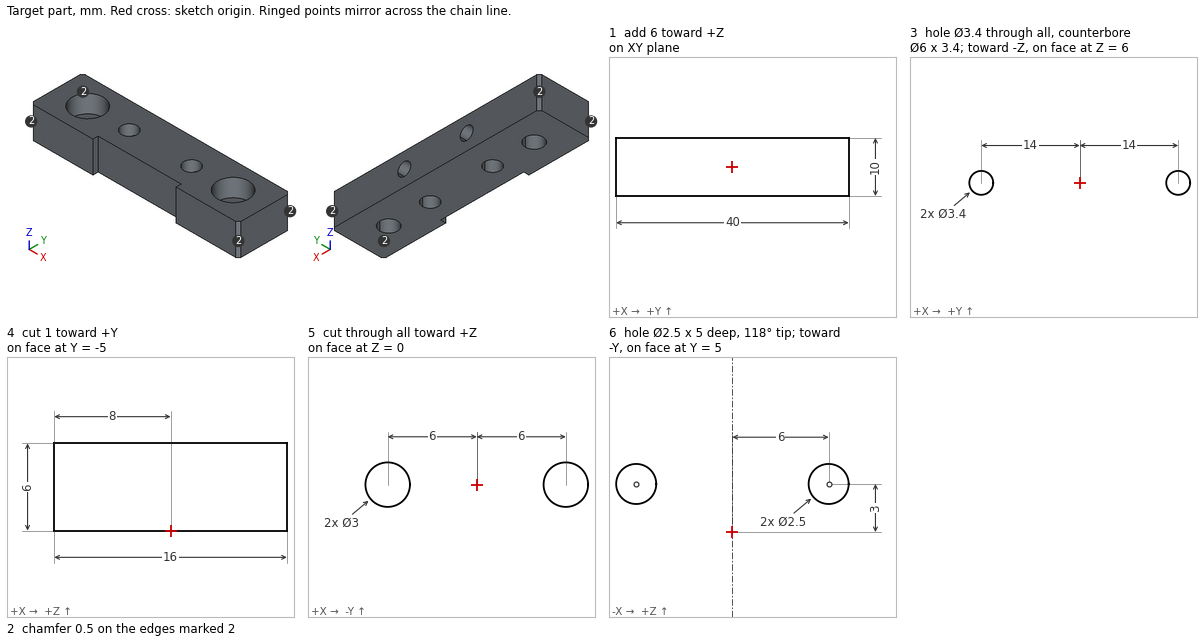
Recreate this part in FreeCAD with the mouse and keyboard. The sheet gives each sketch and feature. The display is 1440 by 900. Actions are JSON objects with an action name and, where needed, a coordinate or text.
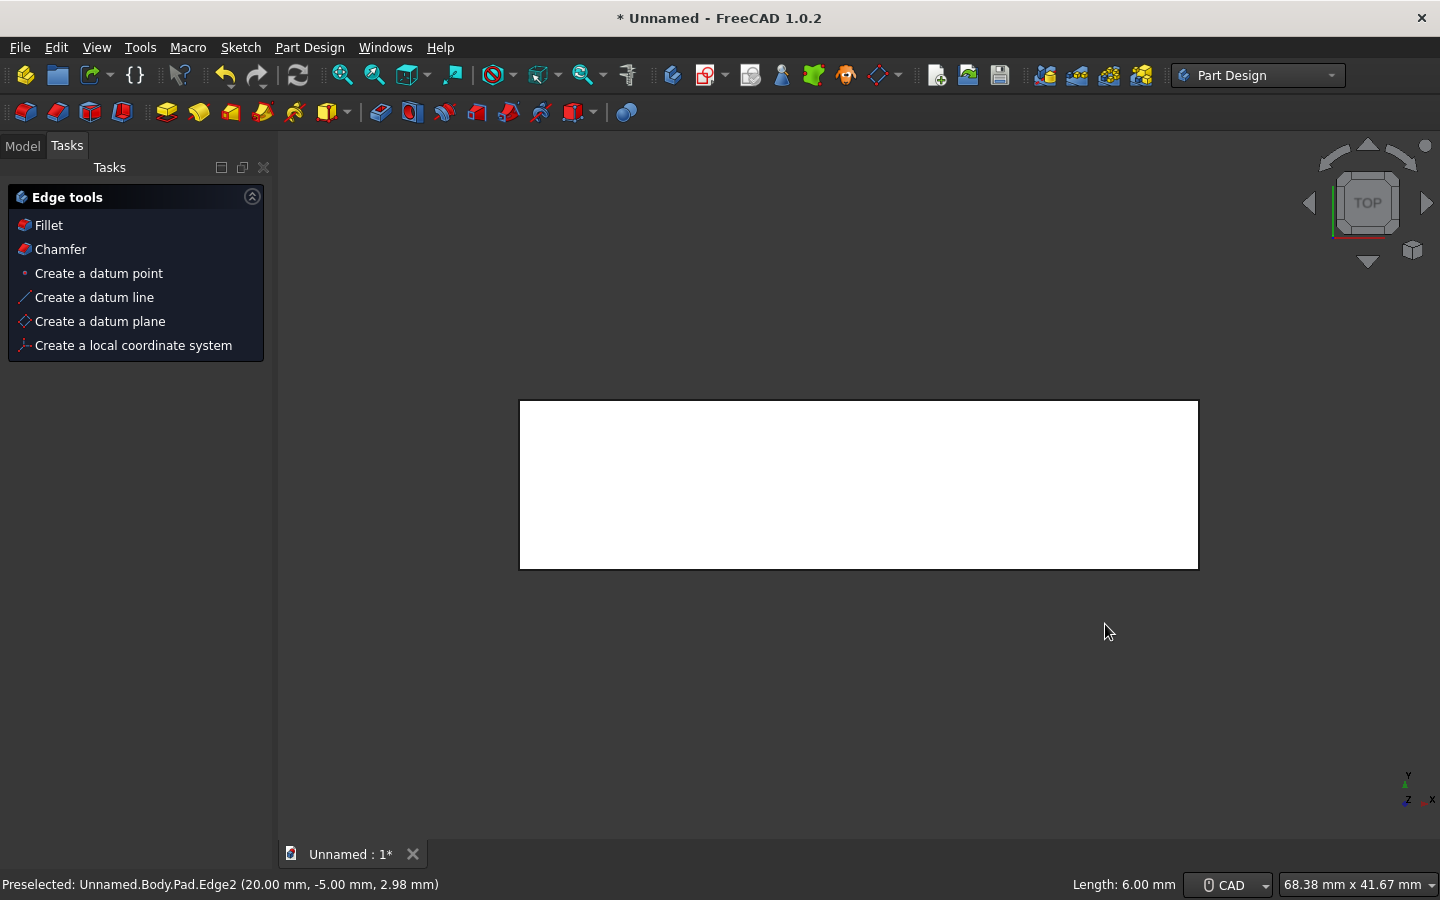
{"action": "key", "text": "1"}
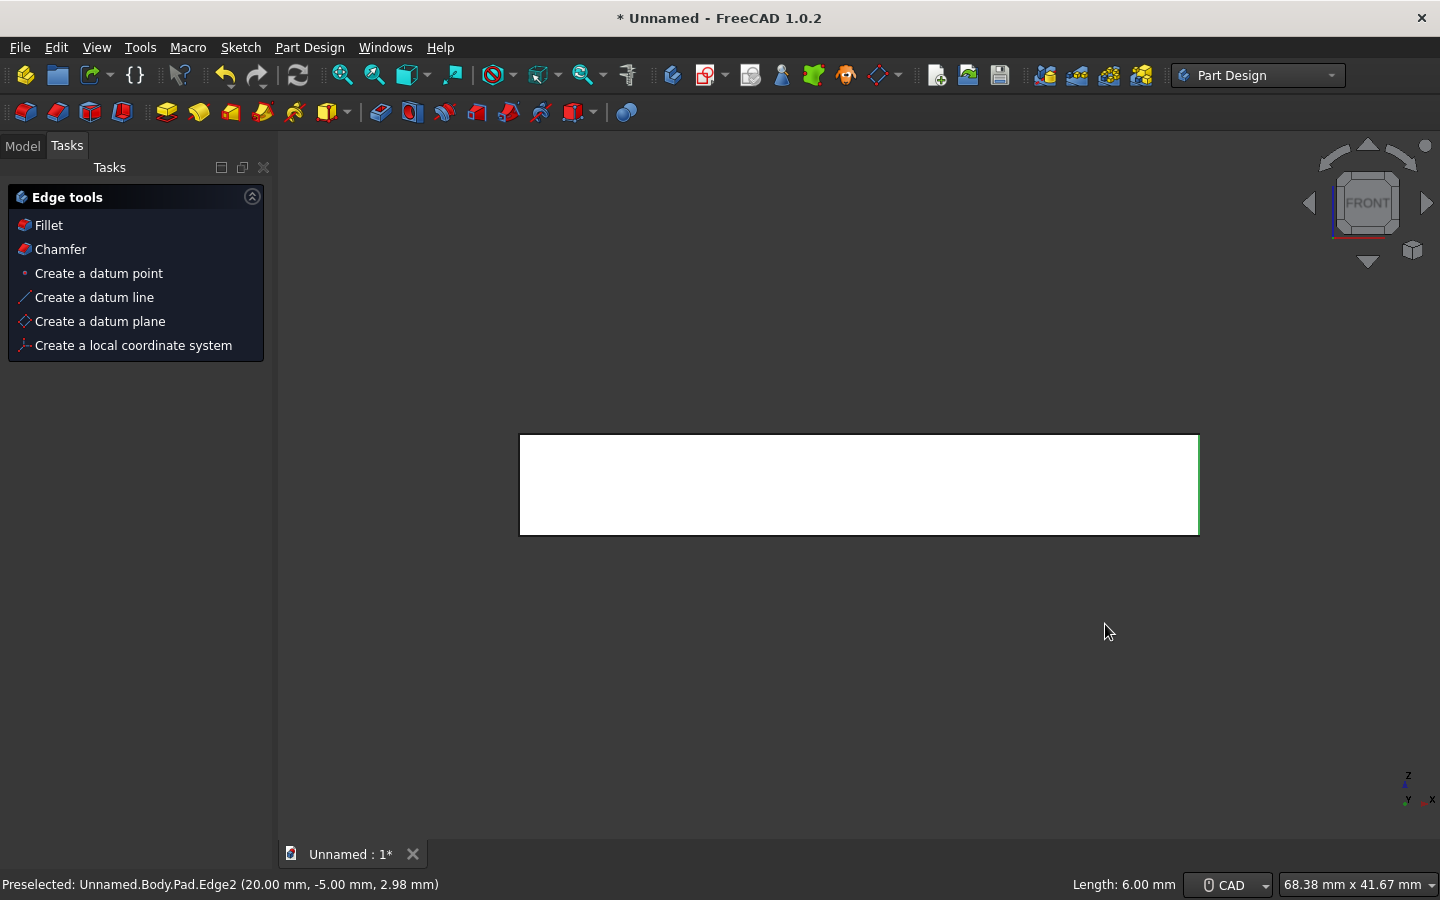
{"action": "left_click", "coordinate": [519, 484], "text": "ctrl"}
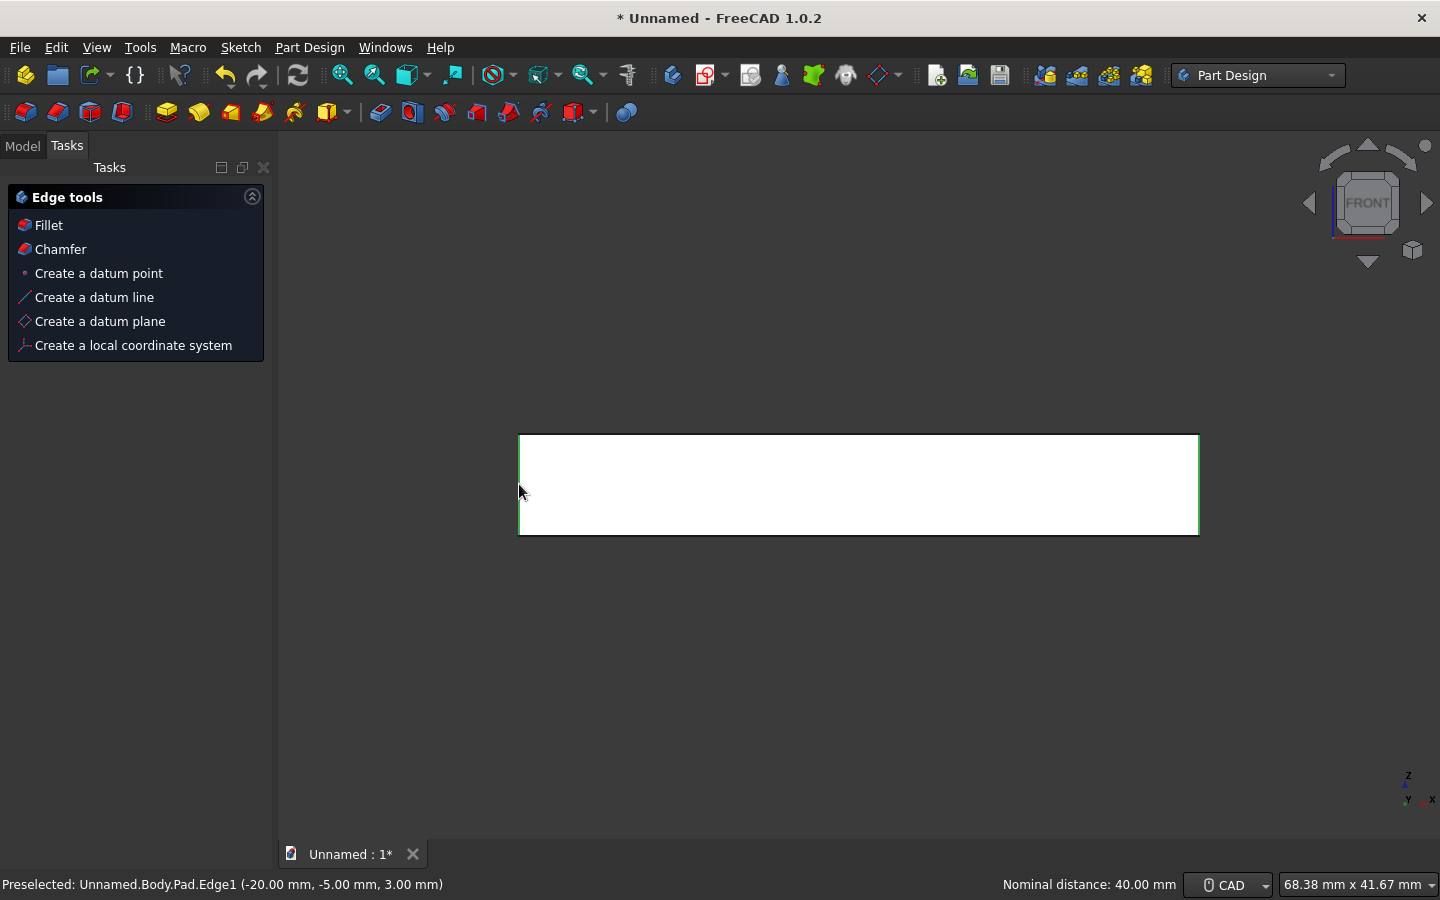
{"action": "key", "text": "3"}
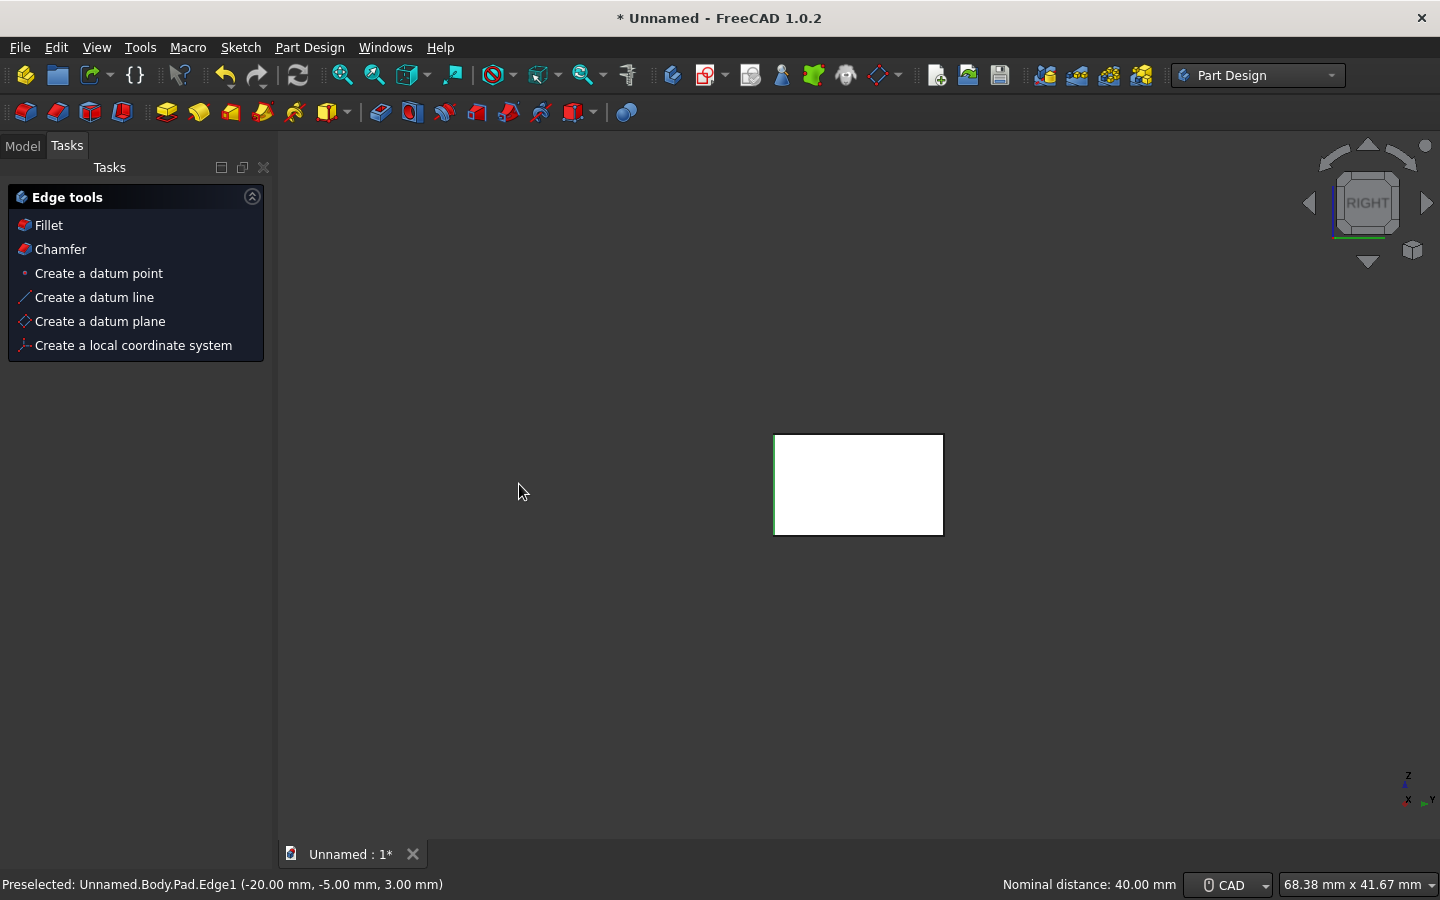
{"action": "left_click", "coordinate": [344, 76]}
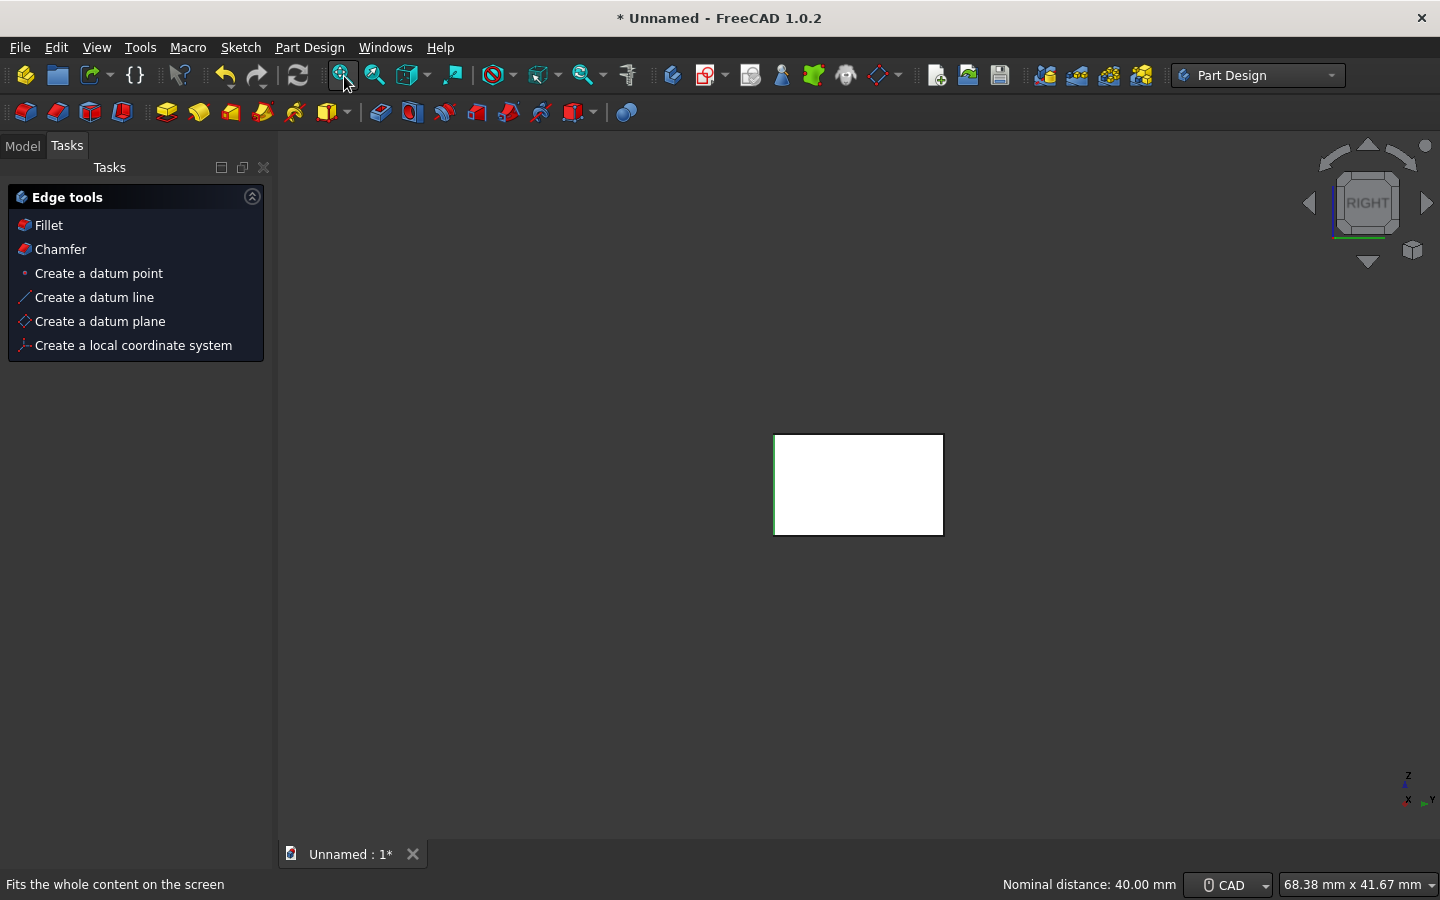
{"action": "left_click", "coordinate": [944, 484], "text": "ctrl"}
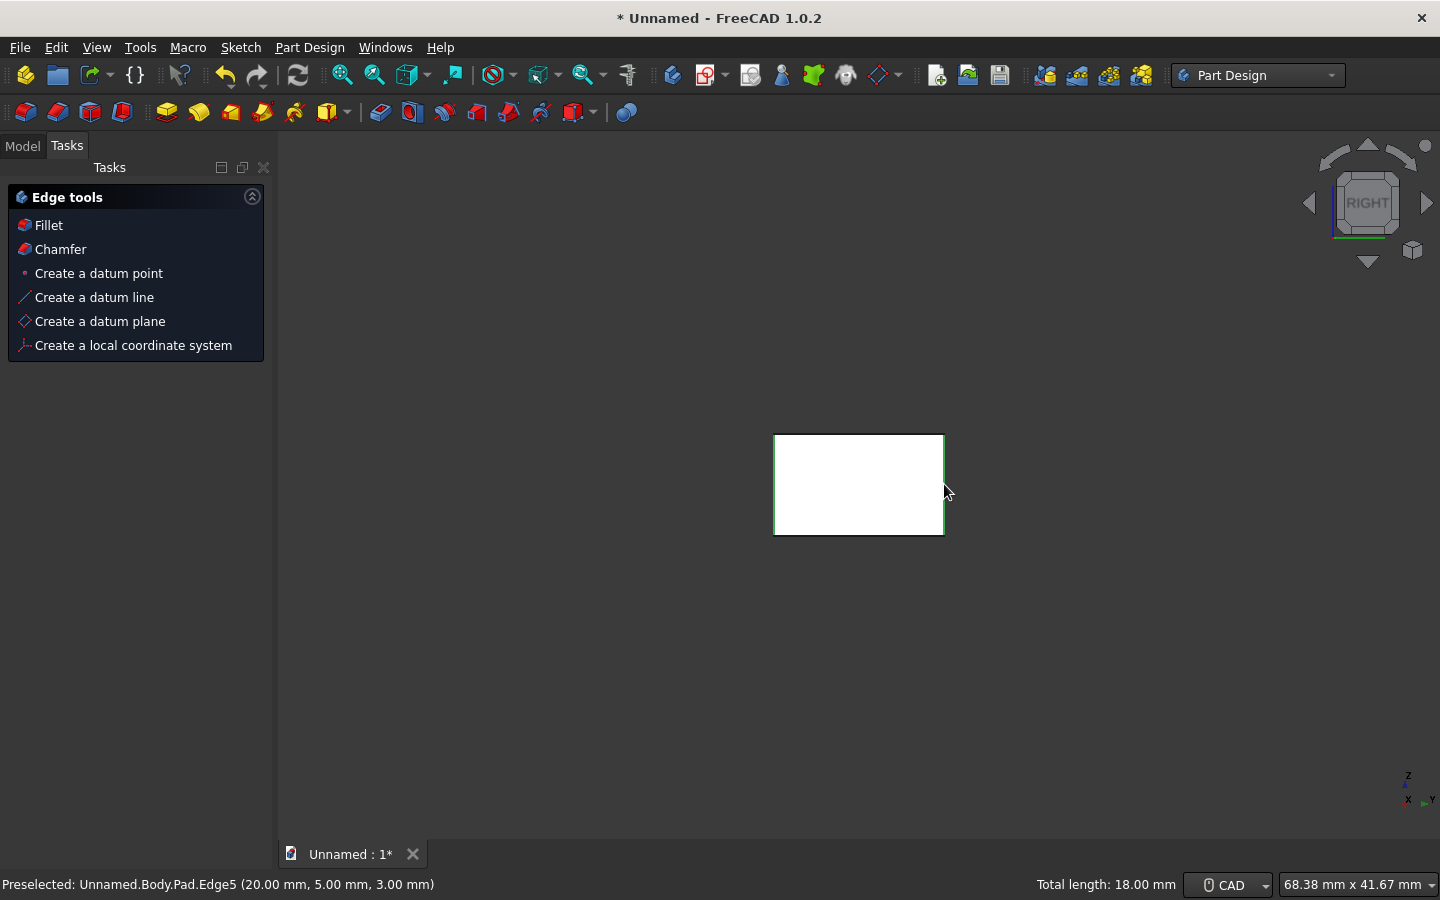
{"action": "key", "text": "5"}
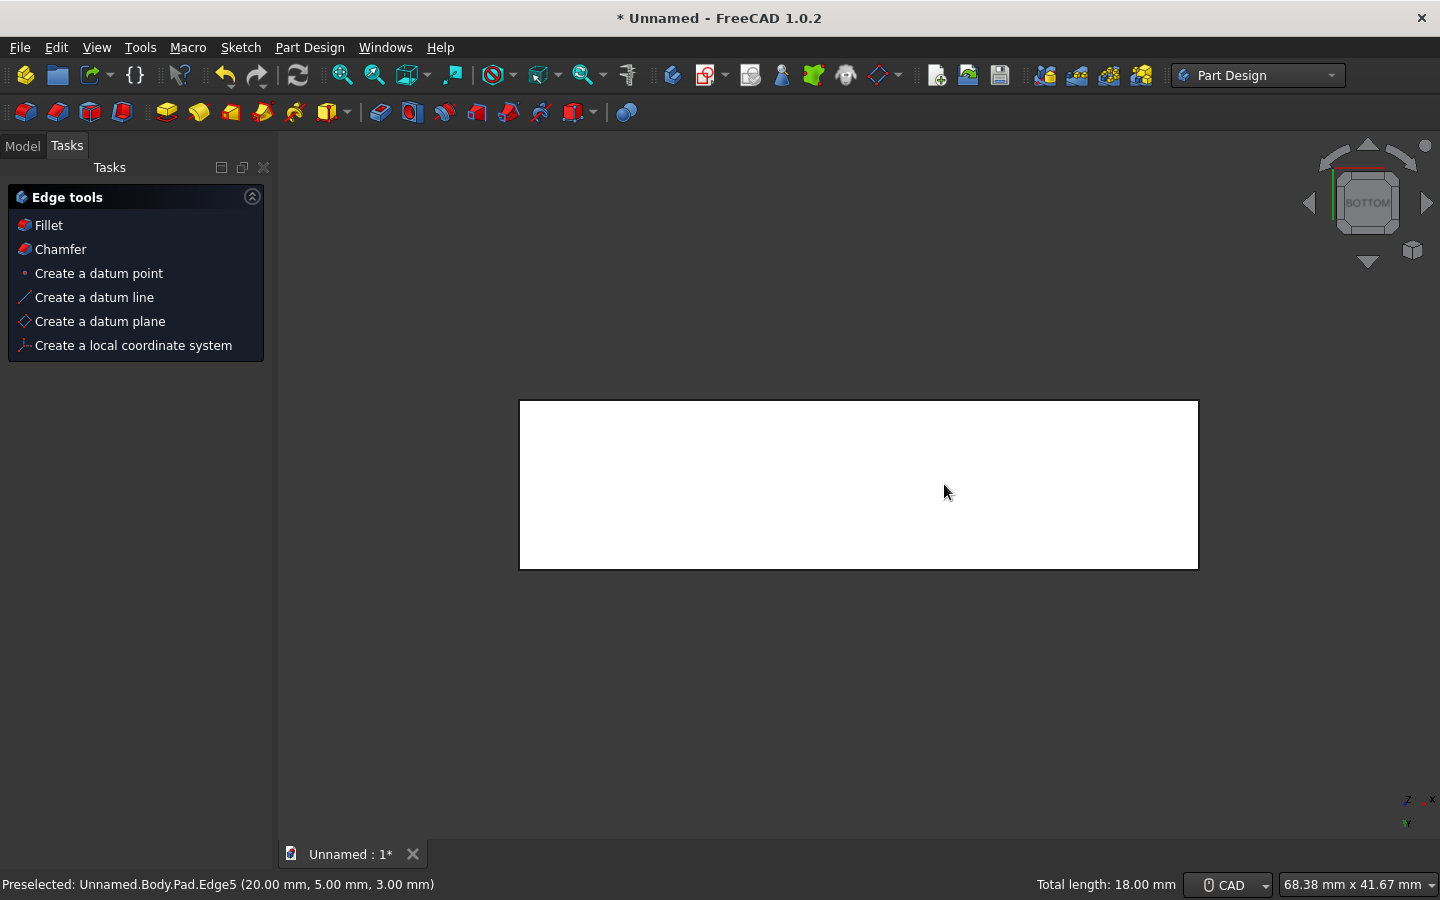
{"action": "key", "text": "4"}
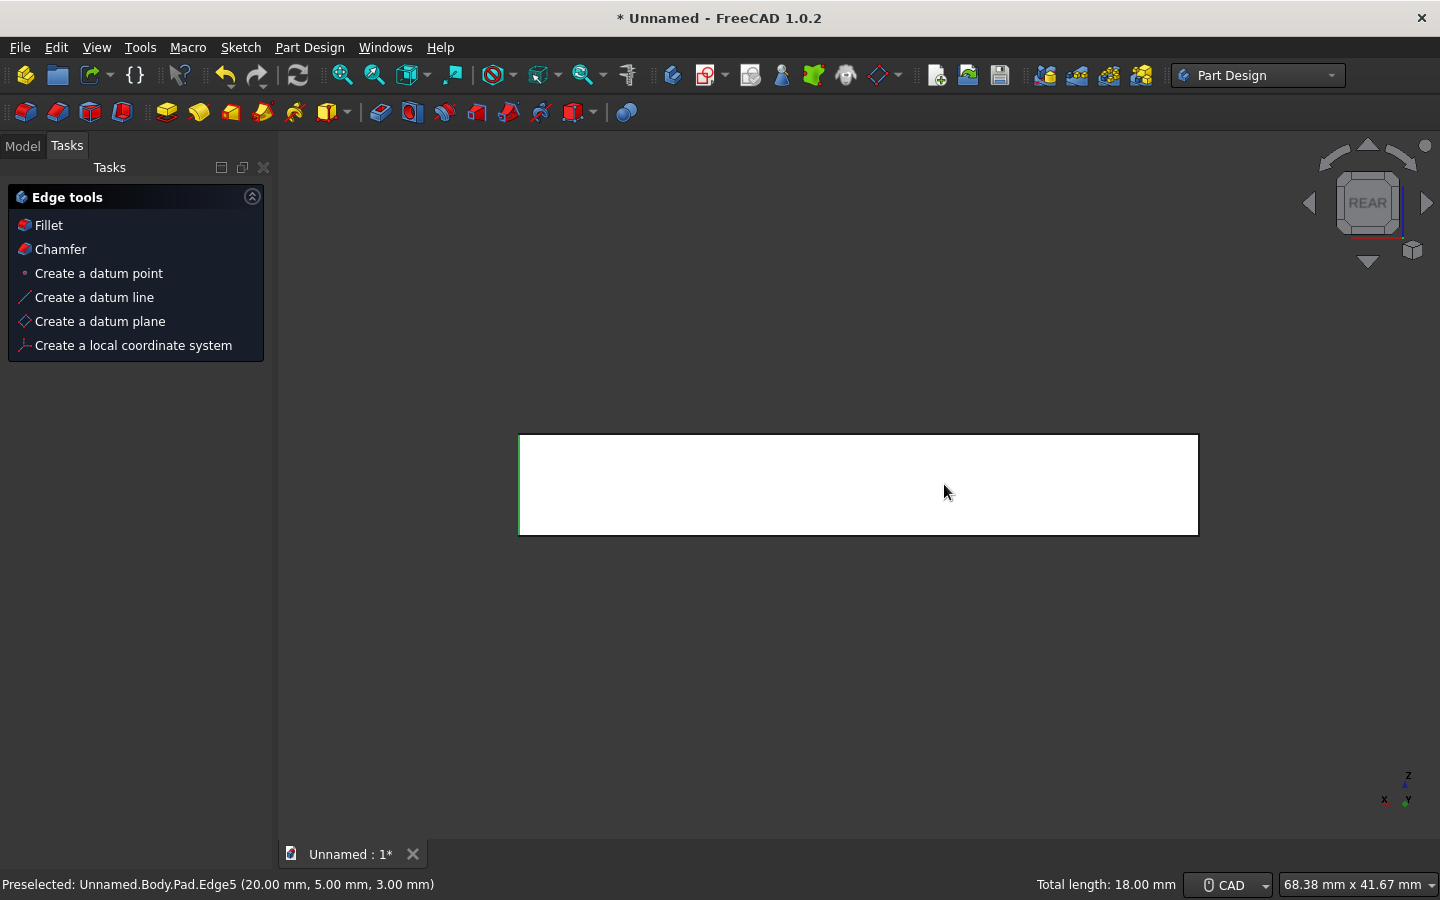
{"action": "left_click", "coordinate": [1199, 484], "text": "ctrl"}